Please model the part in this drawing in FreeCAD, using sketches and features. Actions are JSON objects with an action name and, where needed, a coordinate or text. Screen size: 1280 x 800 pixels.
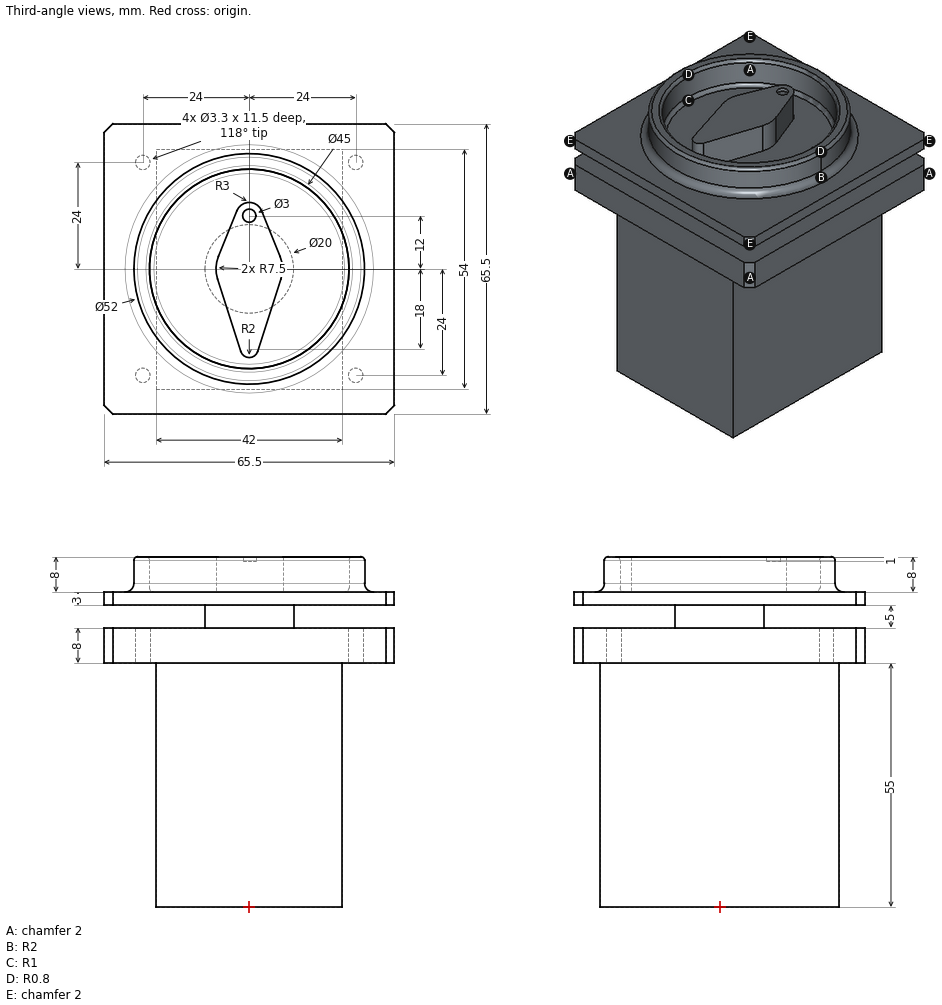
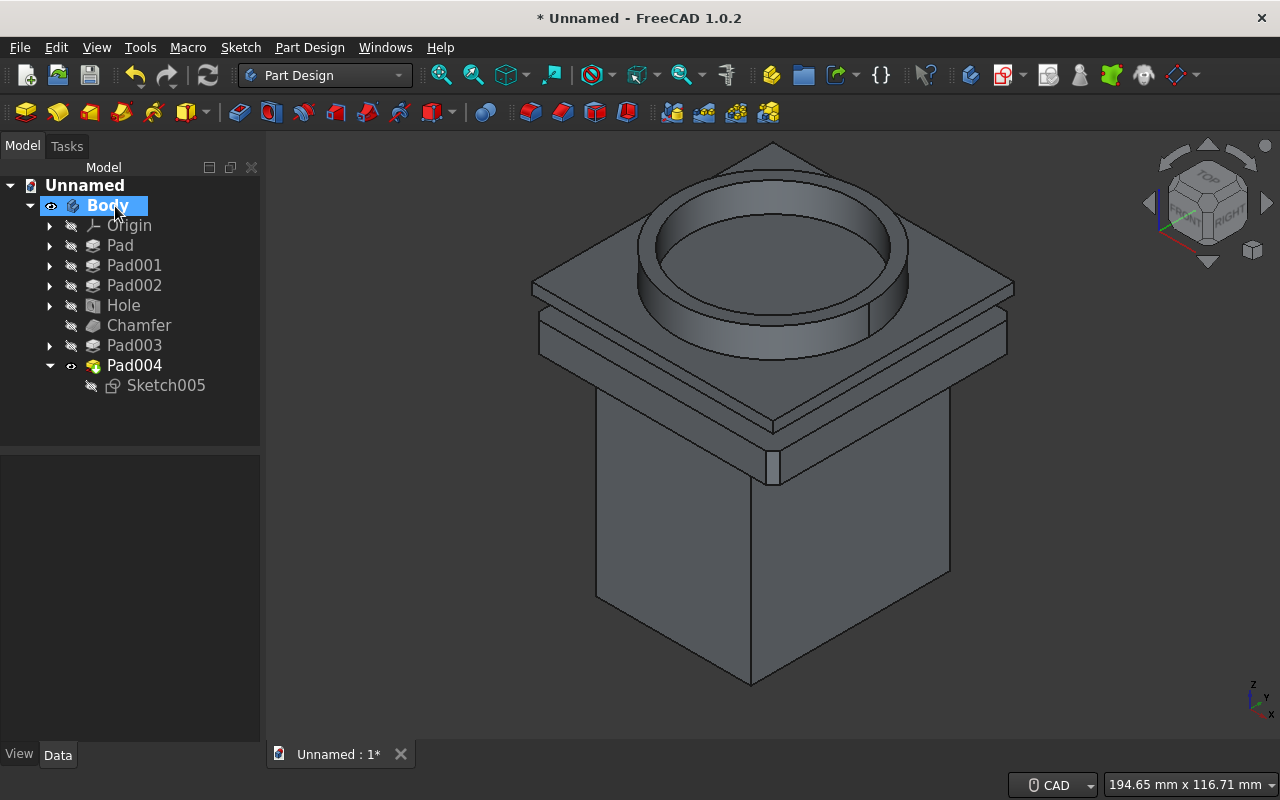
{"action": "left_click", "coordinate": [442, 76]}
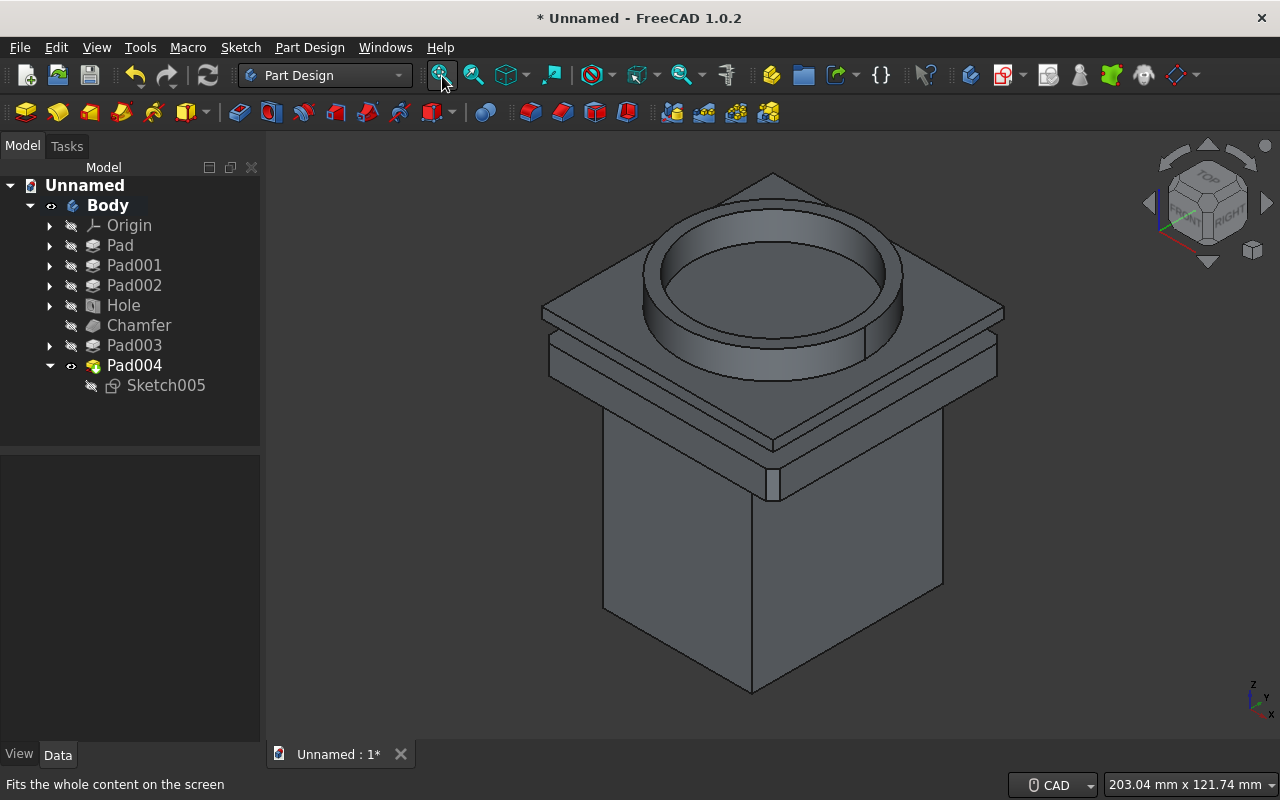
{"action": "left_click", "coordinate": [971, 306]}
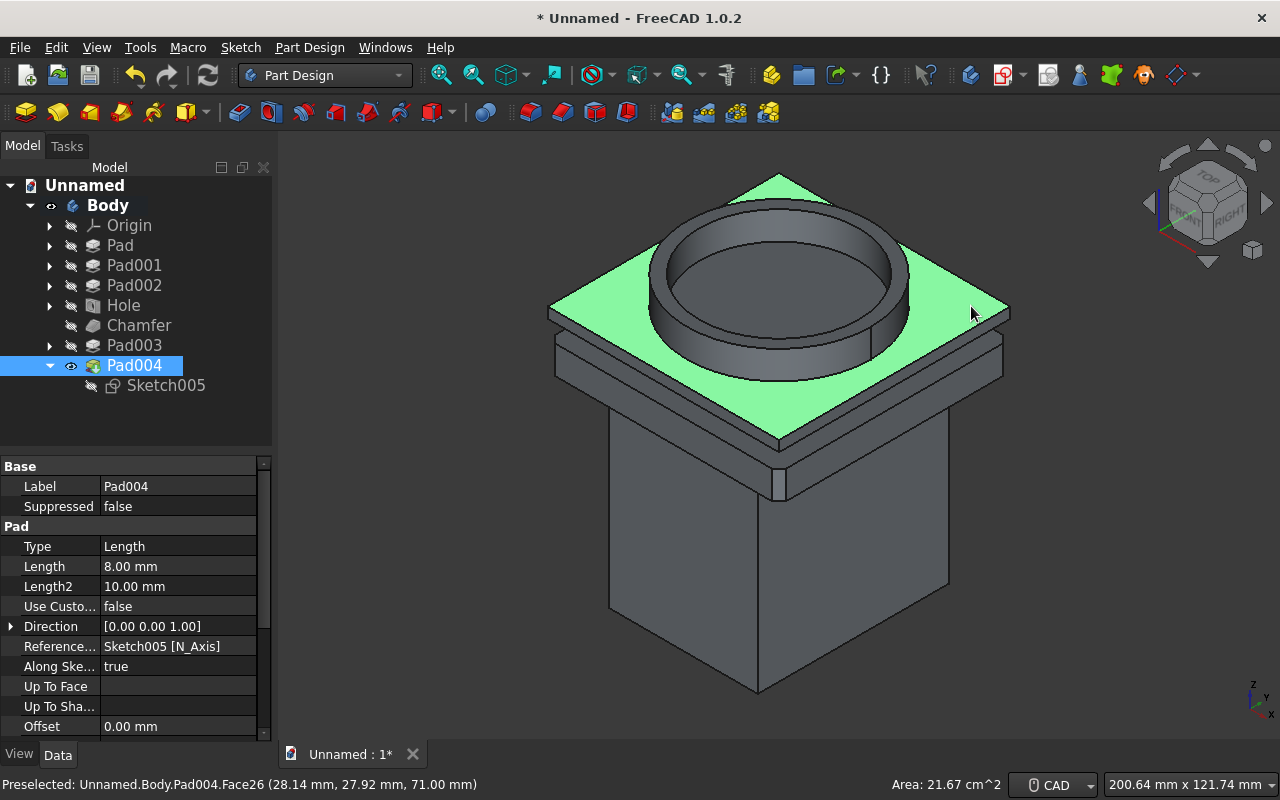
{"action": "left_click", "coordinate": [1004, 76]}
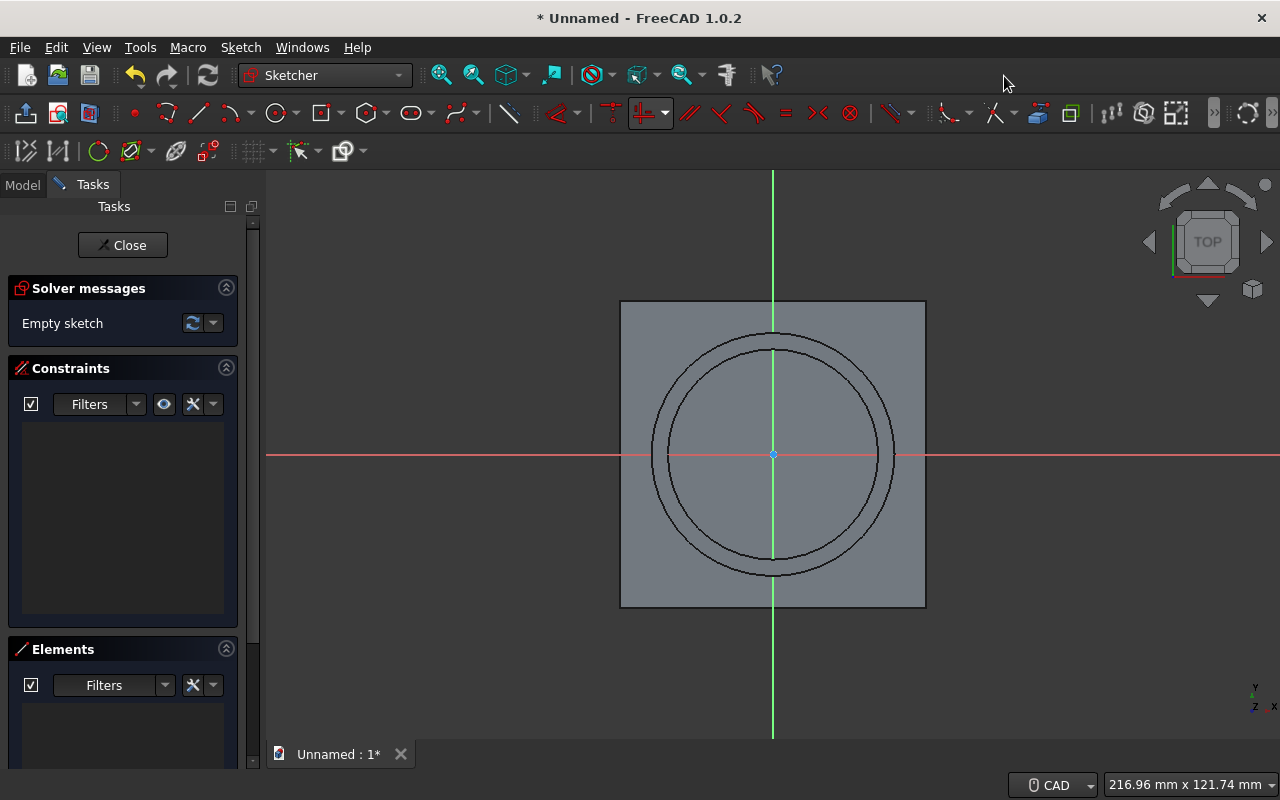
{"action": "scroll", "coordinate": [829, 476], "scroll_direction": "up", "scroll_amount": 4}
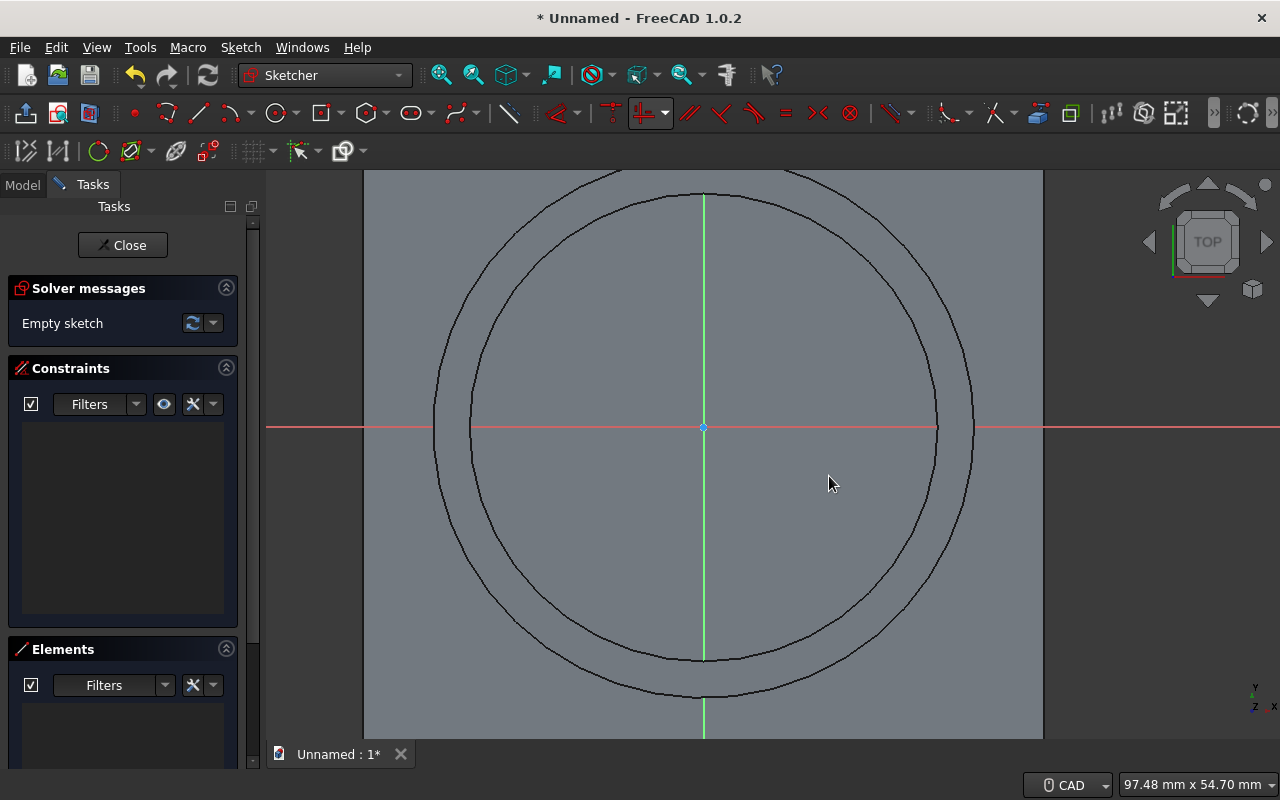
{"action": "left_click", "coordinate": [200, 114]}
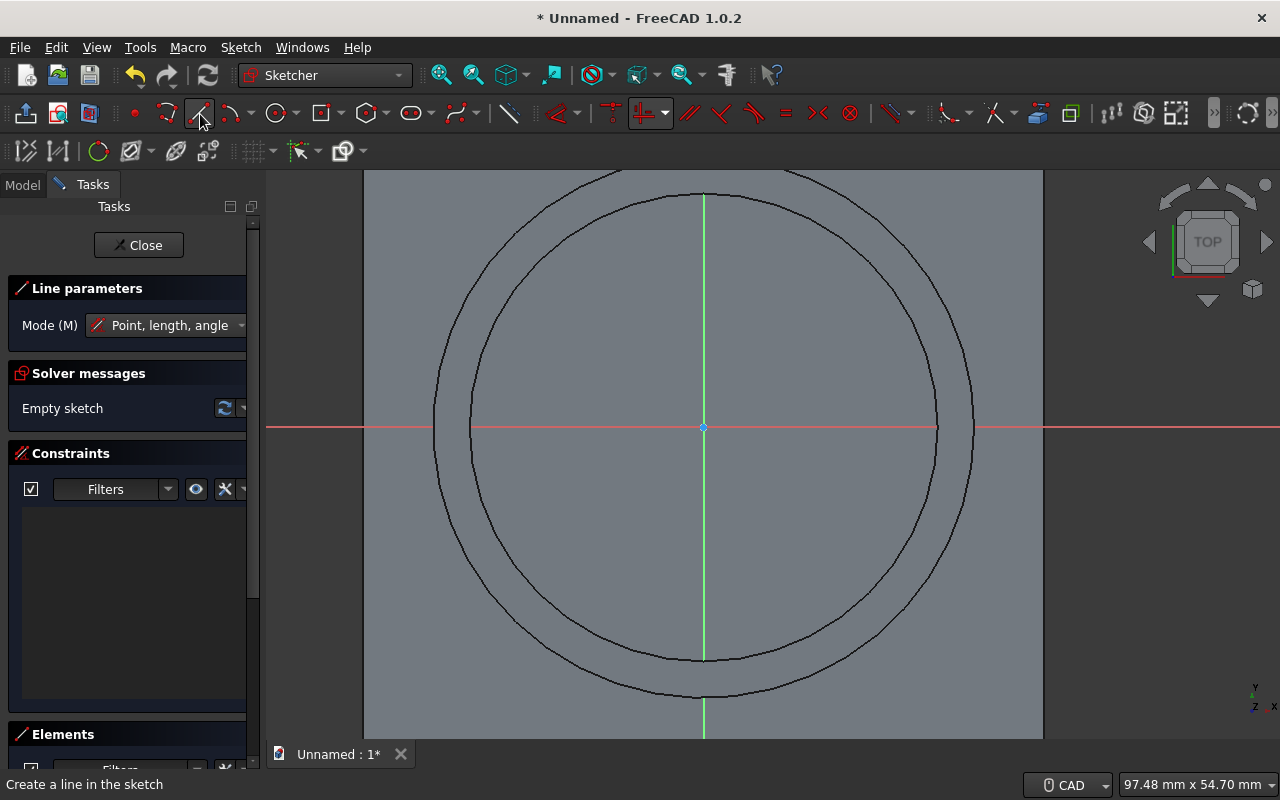
{"action": "left_click", "coordinate": [776, 398]}
{"action": "left_click", "coordinate": [733, 291]}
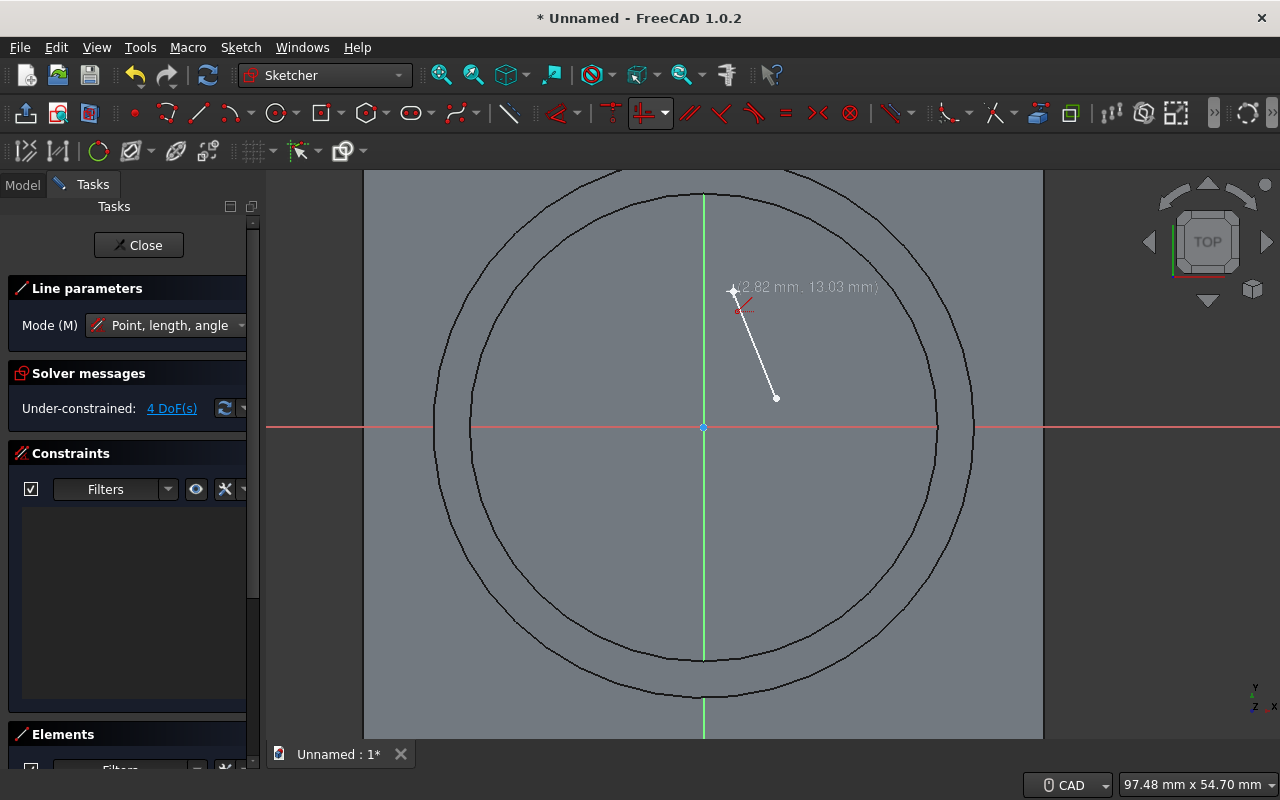
{"action": "left_click", "coordinate": [675, 291]}
{"action": "left_click", "coordinate": [631, 398]}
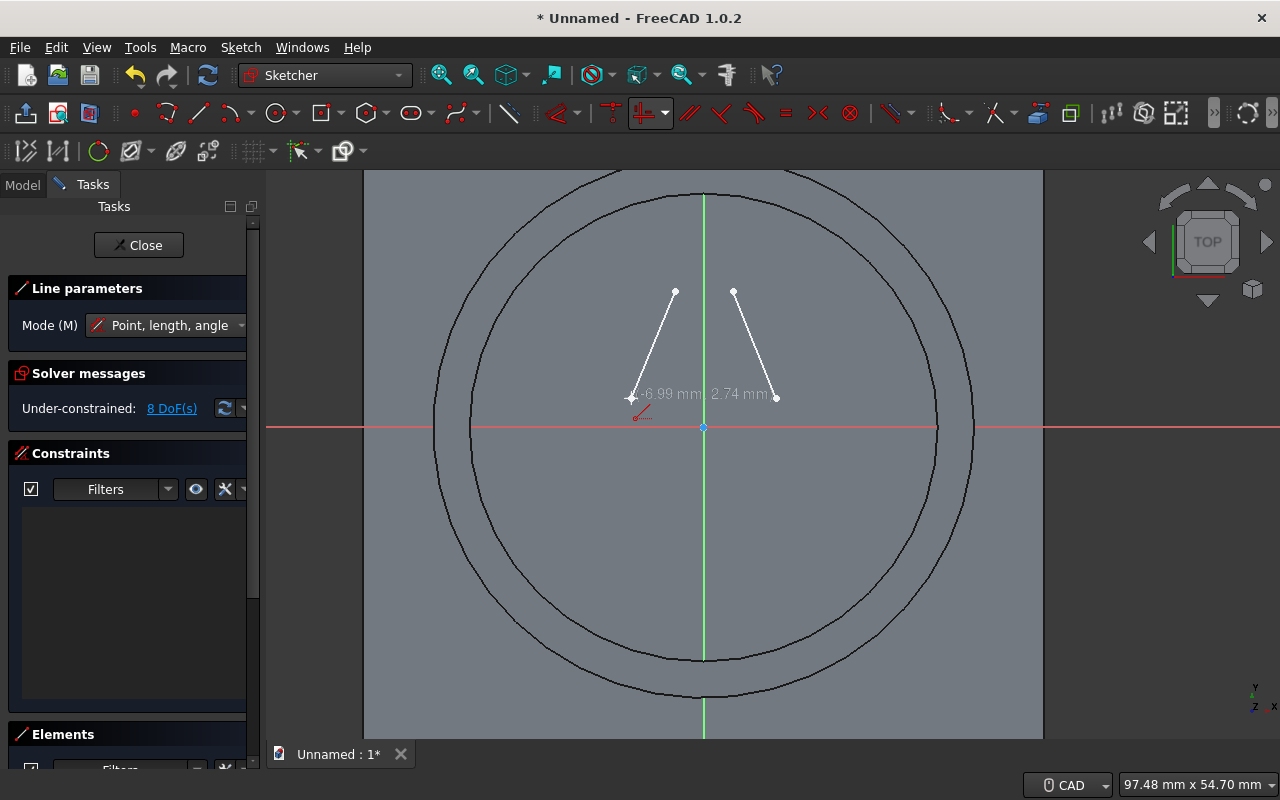
{"action": "left_click", "coordinate": [629, 451]}
{"action": "left_click", "coordinate": [684, 621]}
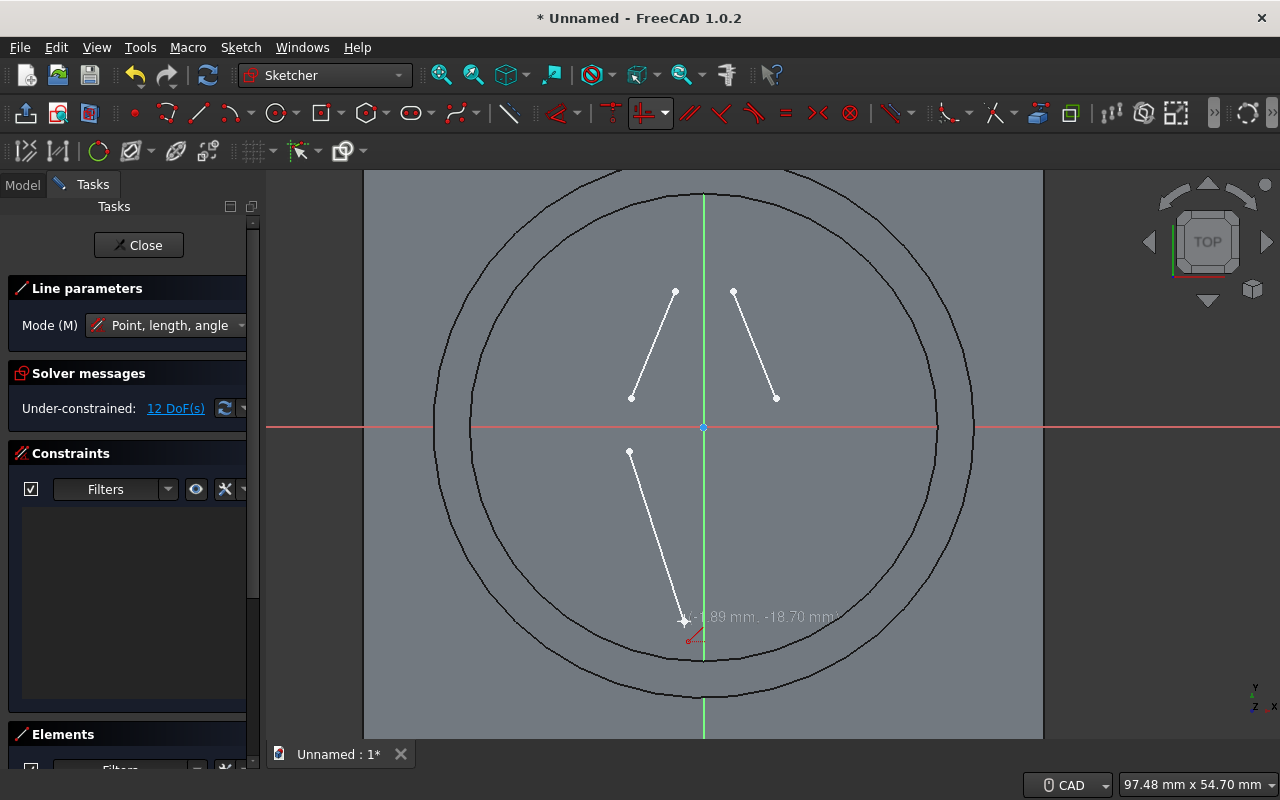
{"action": "left_click", "coordinate": [723, 621]}
{"action": "left_click", "coordinate": [778, 451]}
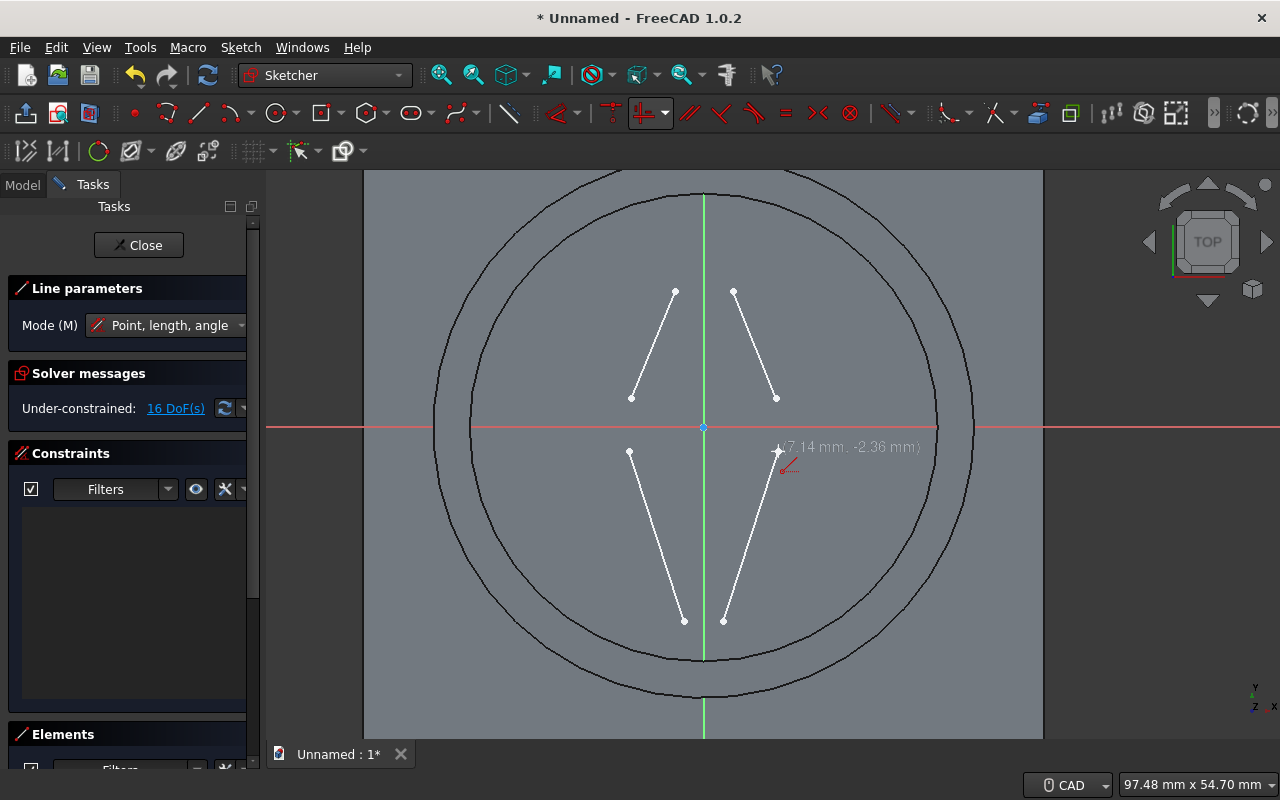
{"action": "left_click", "coordinate": [254, 114]}